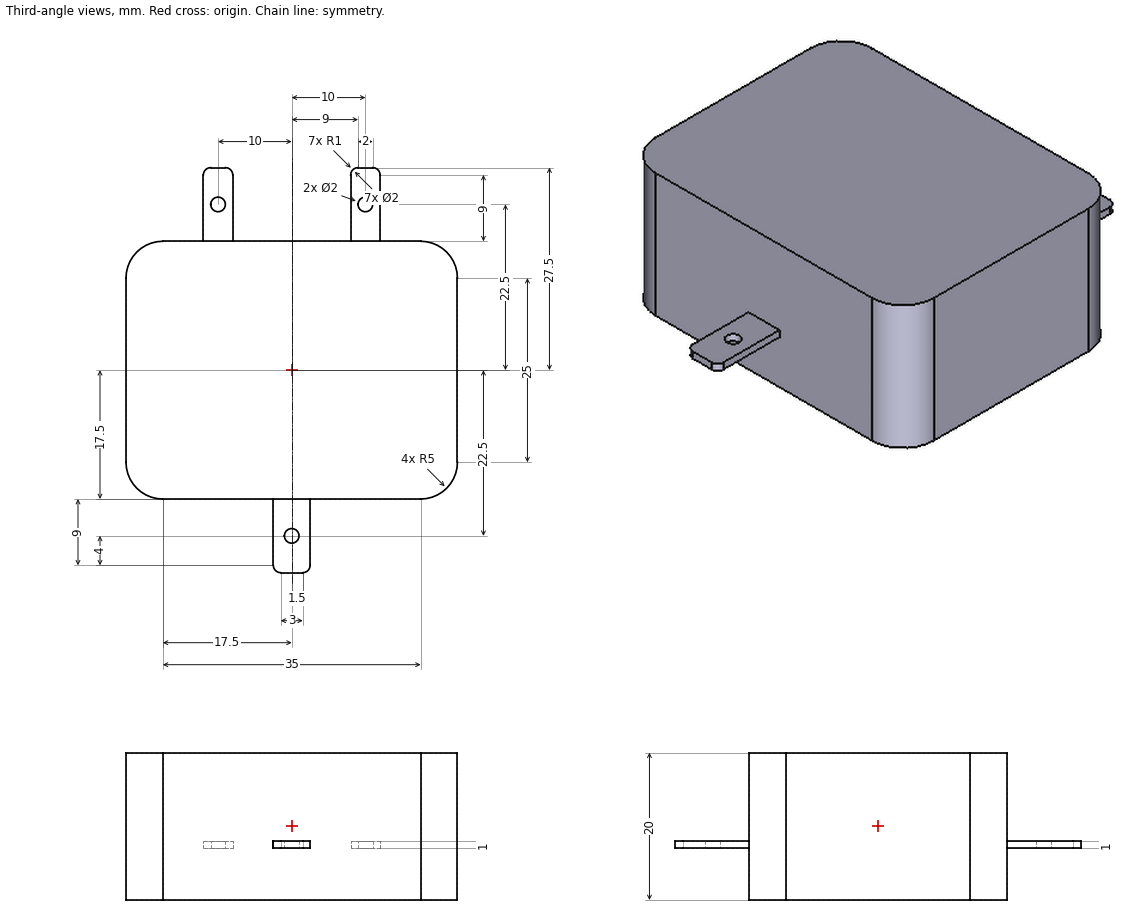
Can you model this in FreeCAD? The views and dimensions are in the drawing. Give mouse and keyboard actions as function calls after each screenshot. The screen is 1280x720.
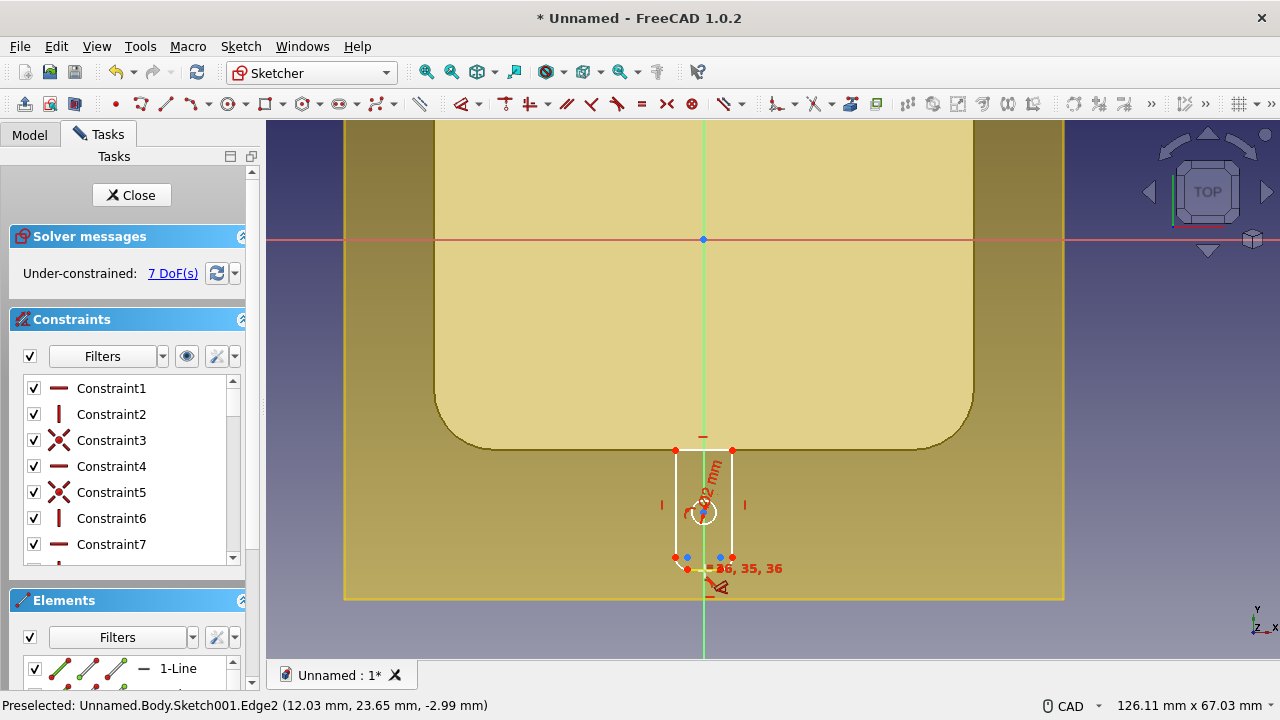
click(704, 569)
click(690, 603)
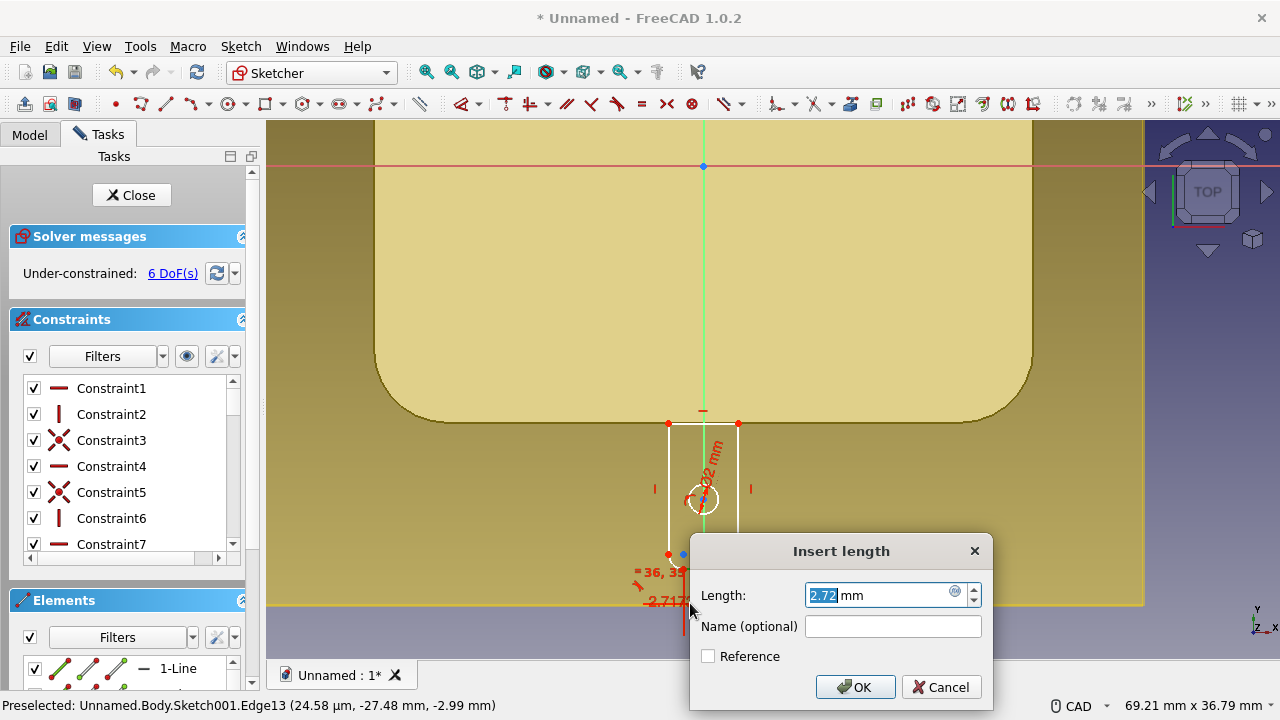
text(3)
key(Return)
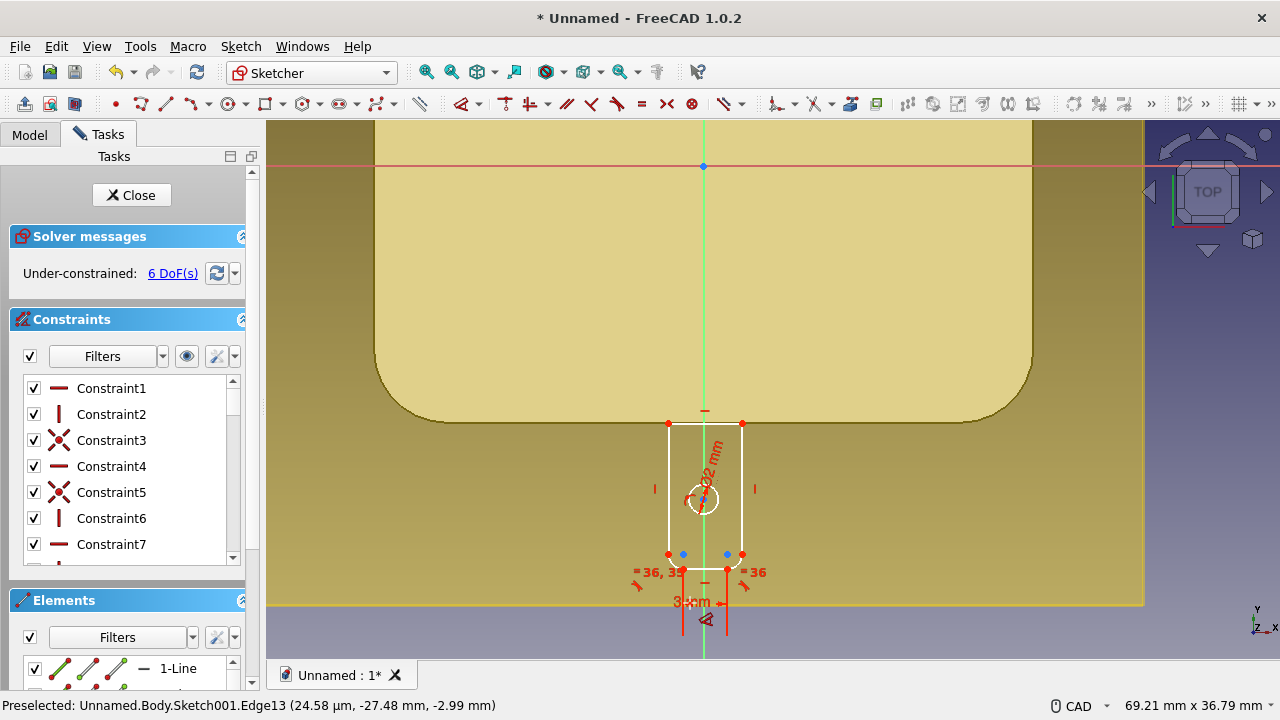
click(669, 515)
click(635, 489)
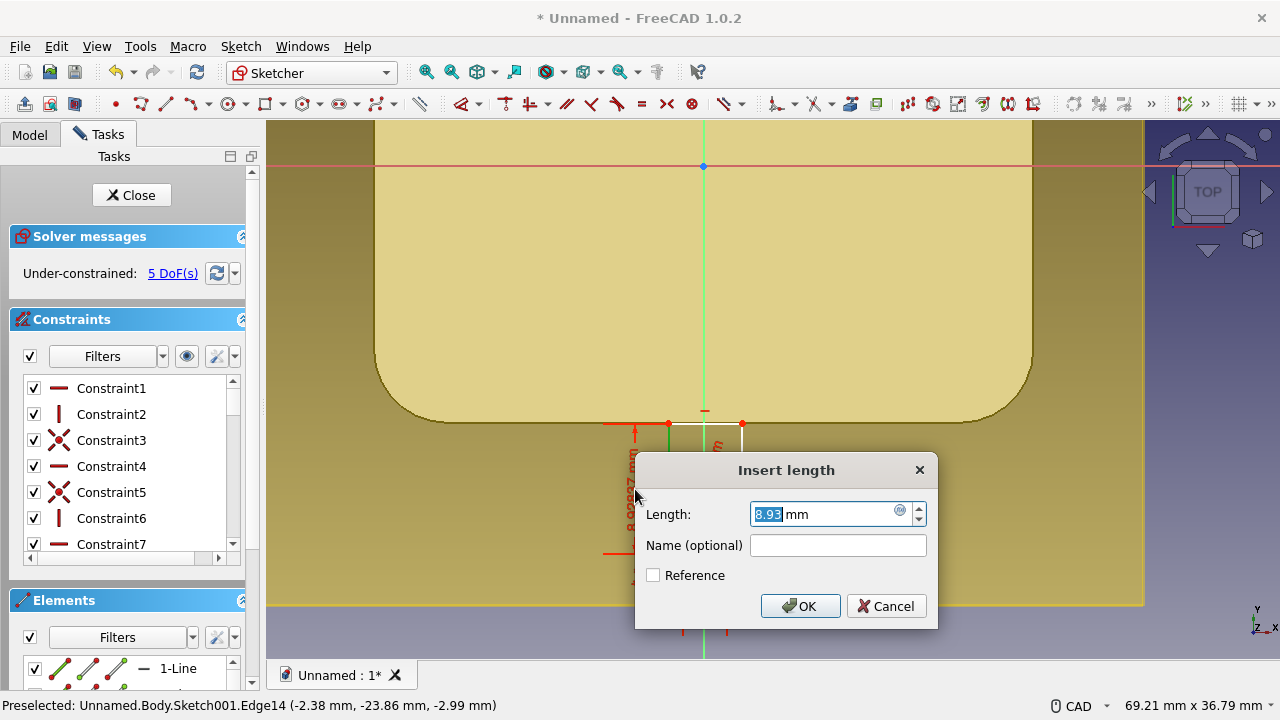
text(9)
key(Return)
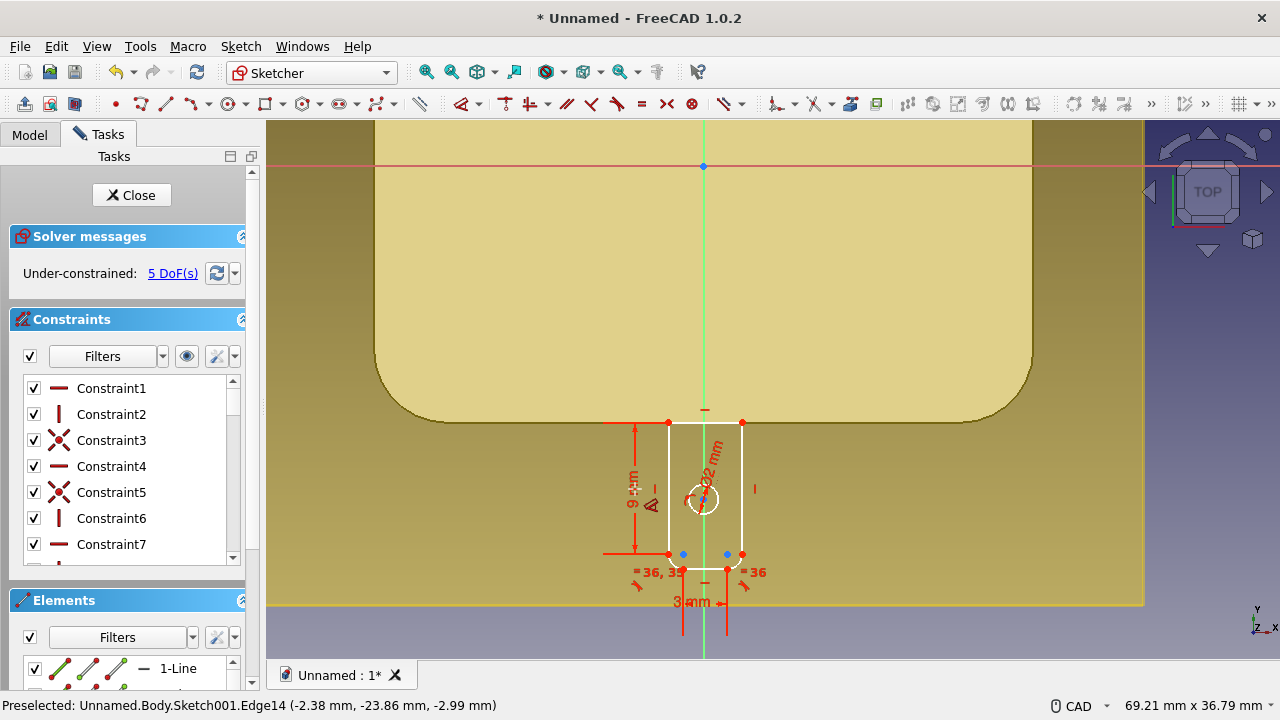
scroll(705, 572, down, 4)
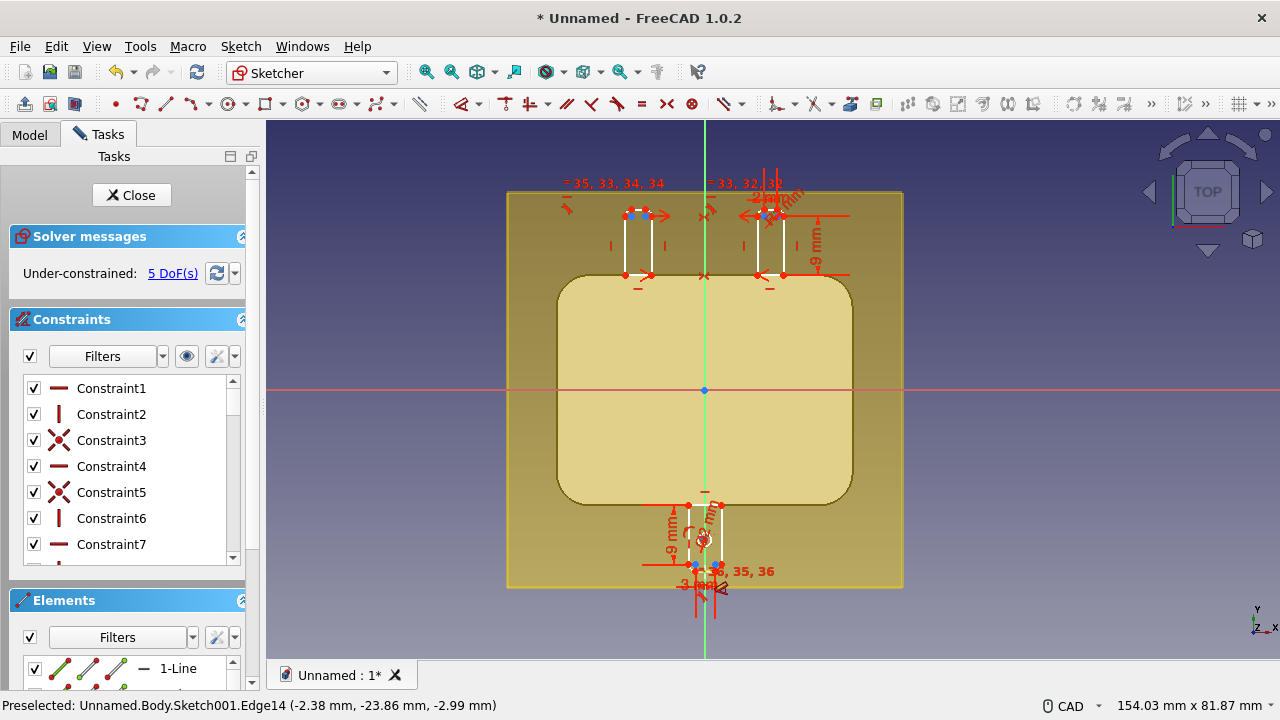
scroll(764, 210, up, 4)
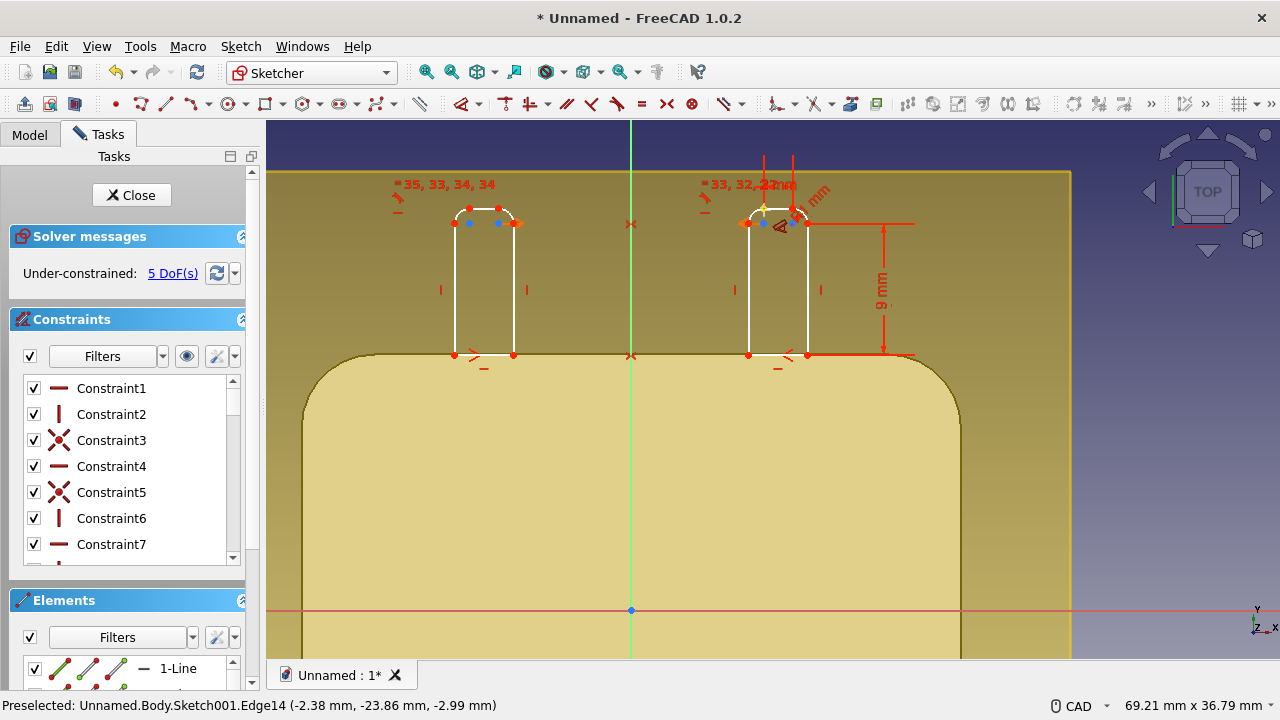
click(764, 209)
click(697, 175)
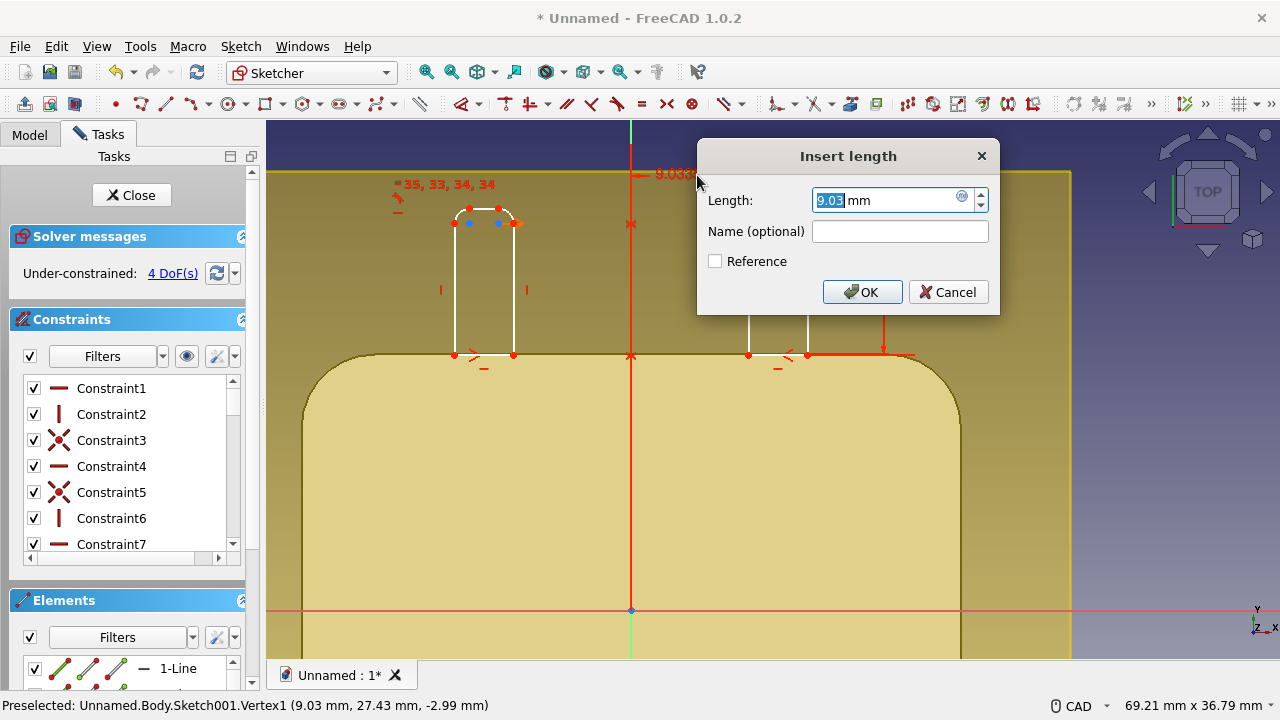
text(9)
key(Return)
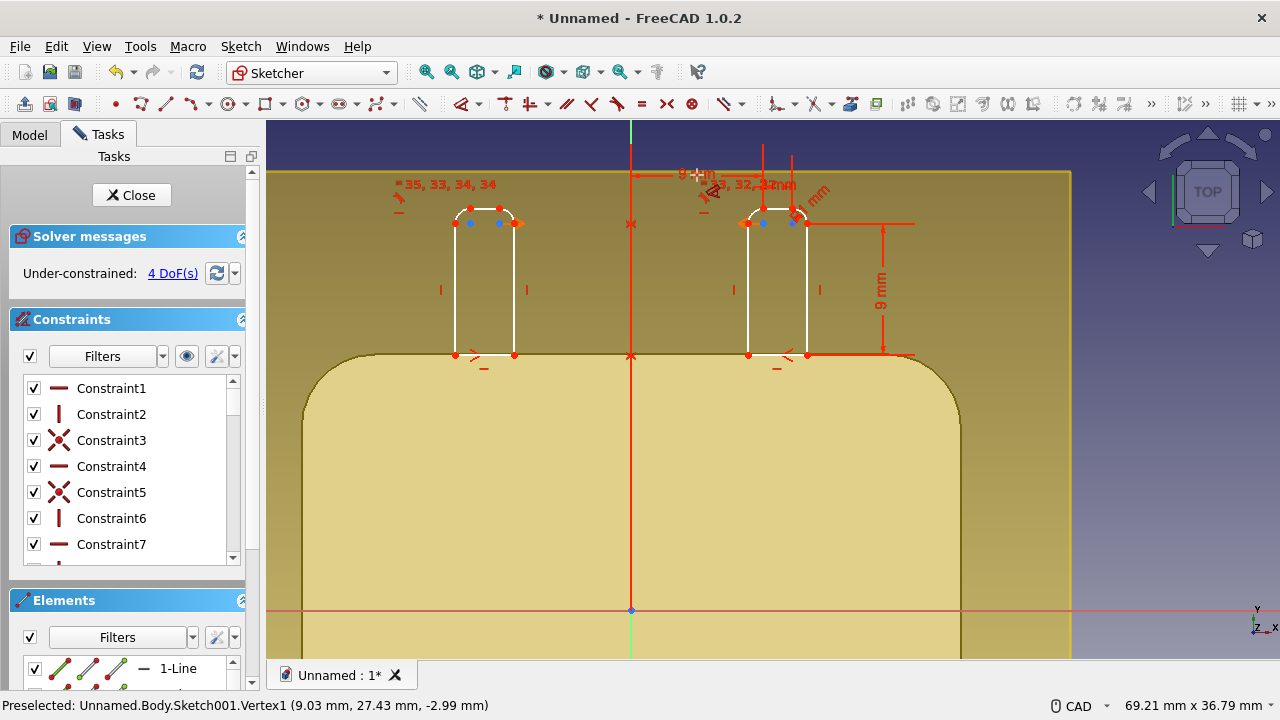
scroll(764, 209, down, 4)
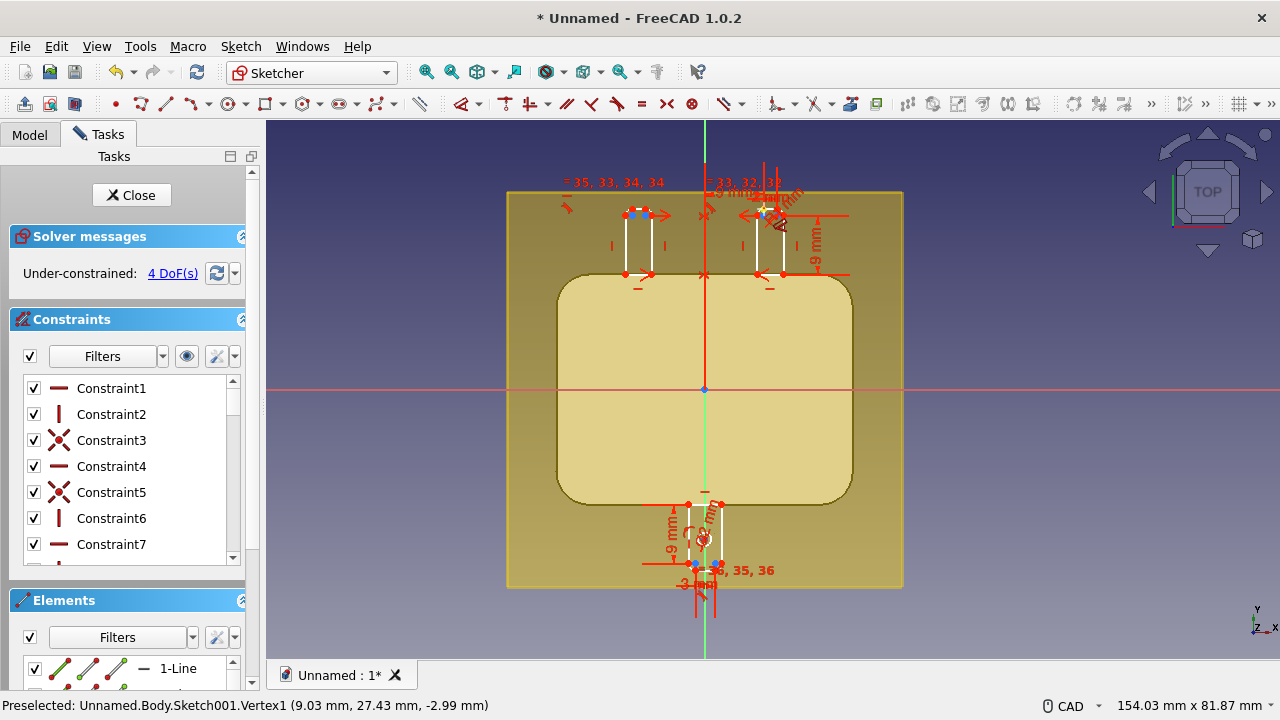
scroll(689, 564, up, 4)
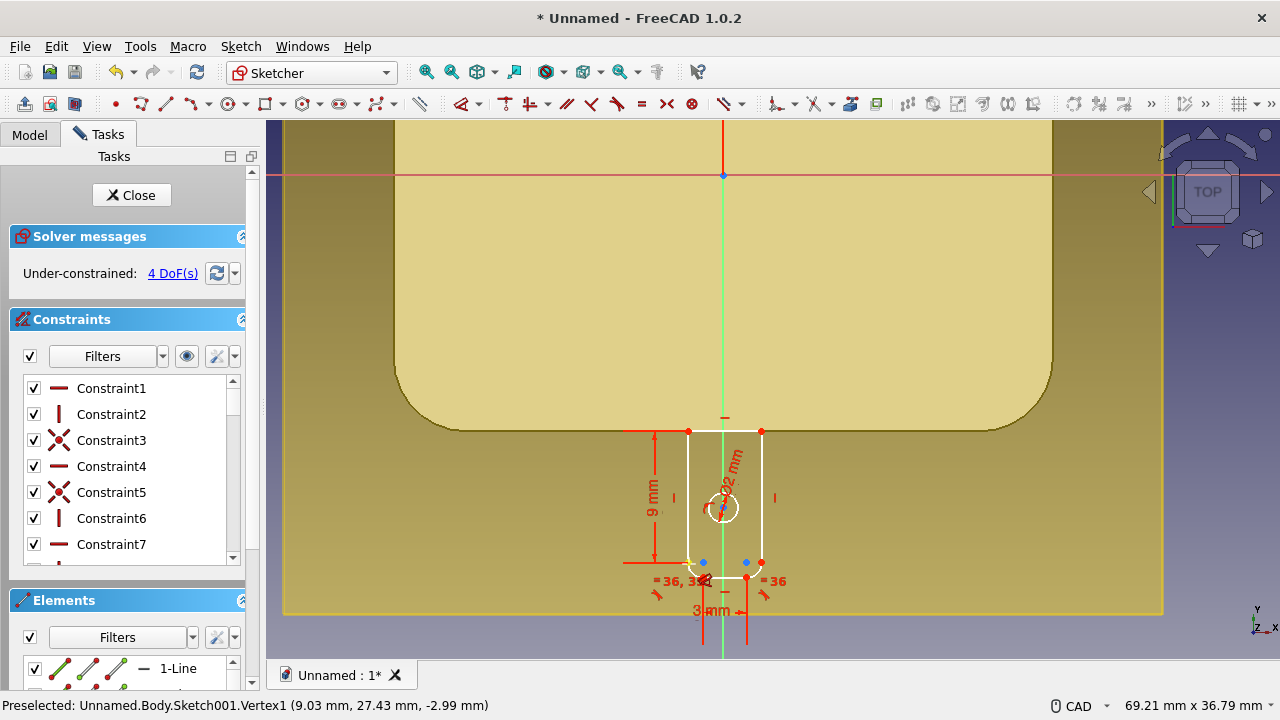
click(688, 563)